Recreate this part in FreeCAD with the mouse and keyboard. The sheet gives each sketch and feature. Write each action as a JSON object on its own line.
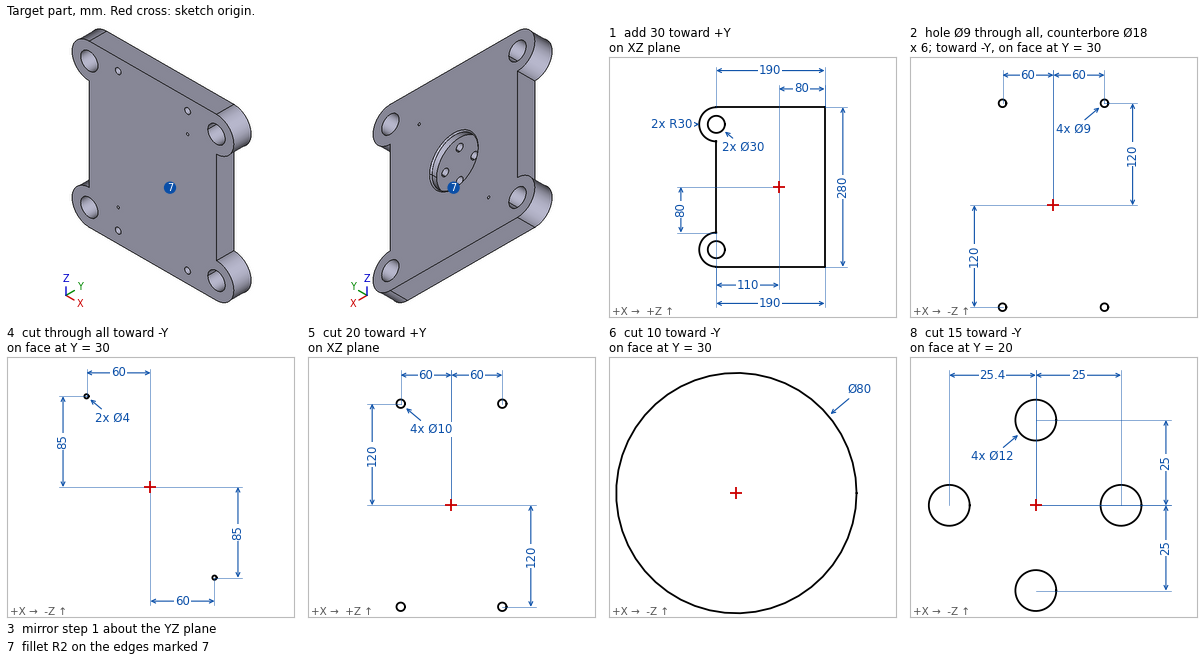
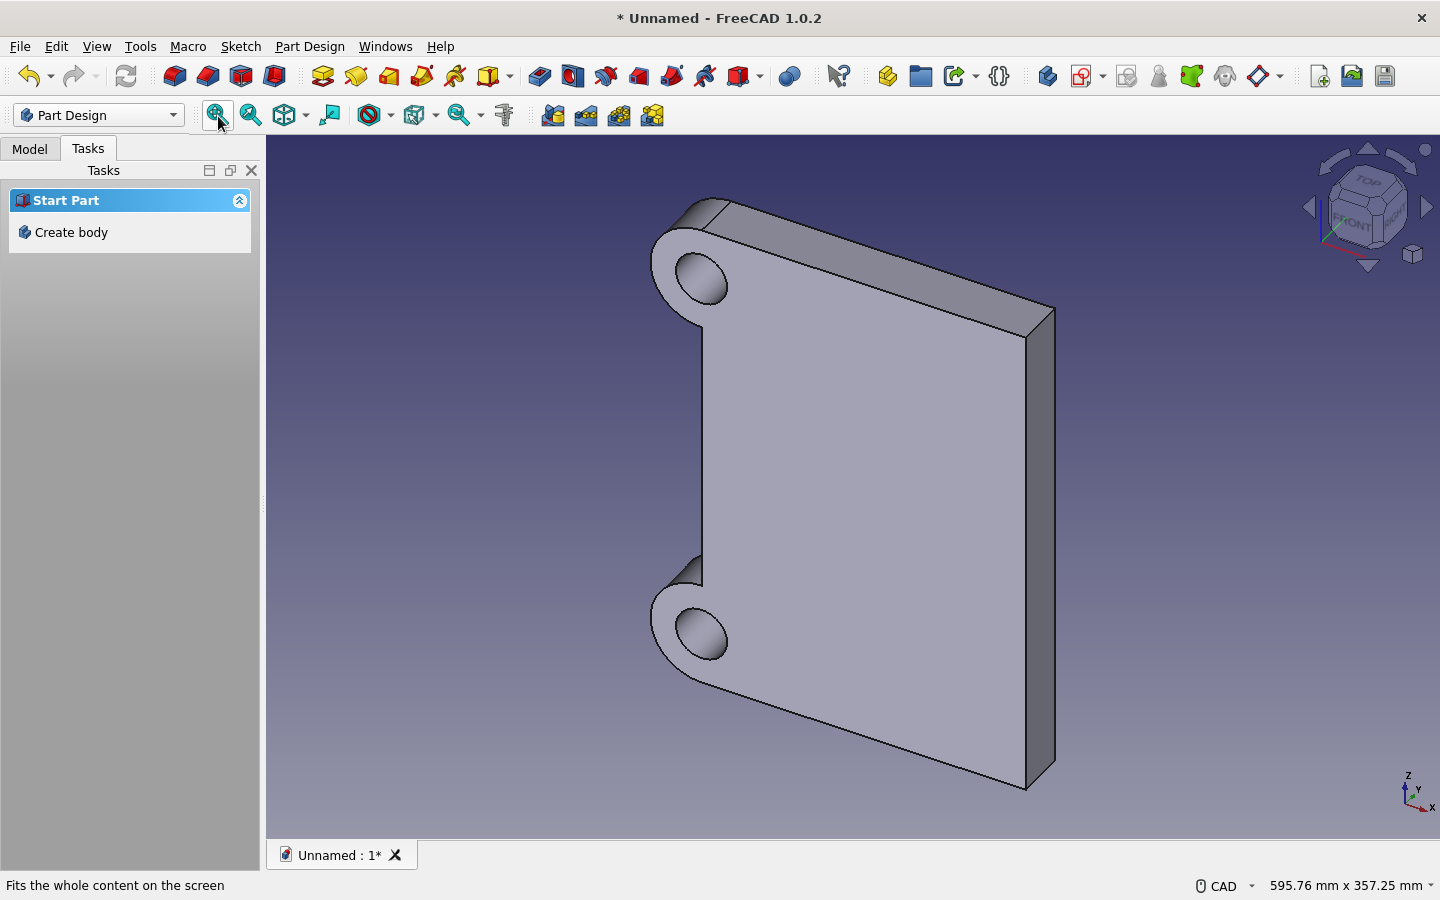
{"action": "key", "text": "4"}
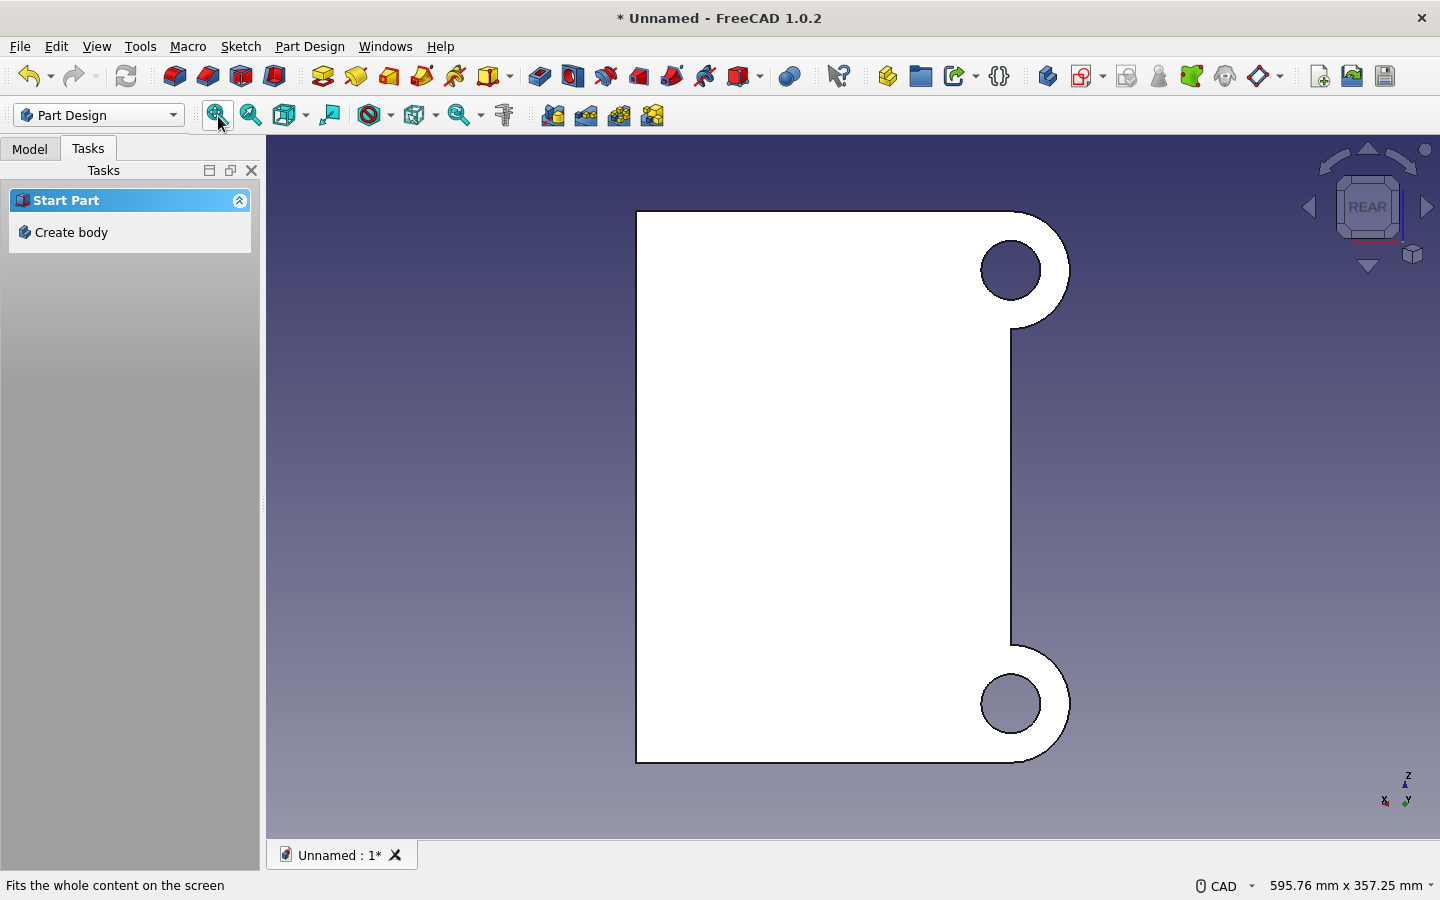
{"action": "left_click", "coordinate": [853, 407]}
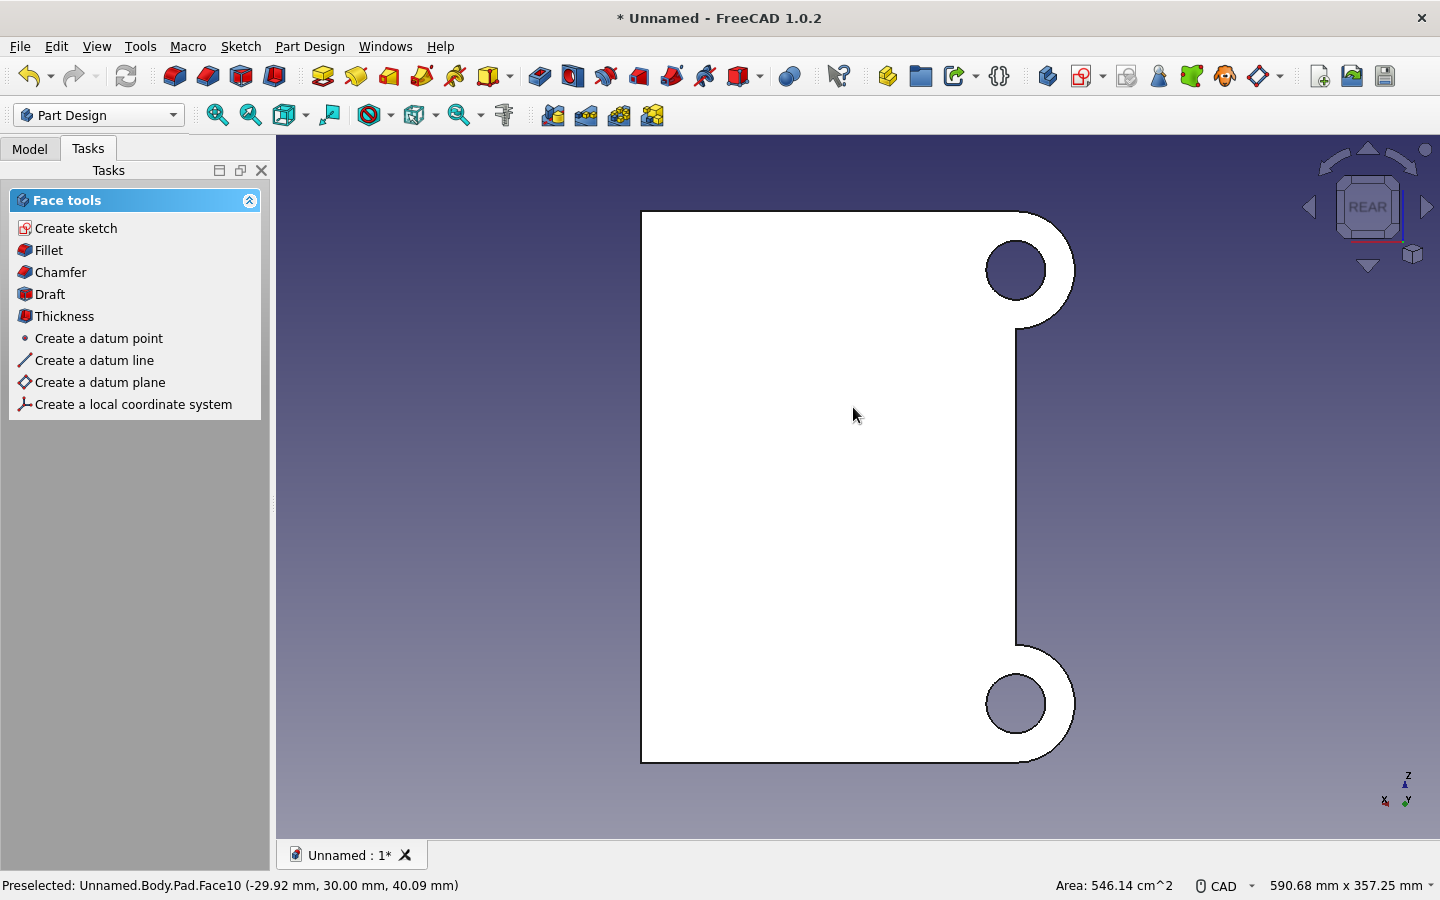
{"action": "left_click", "coordinate": [1080, 76]}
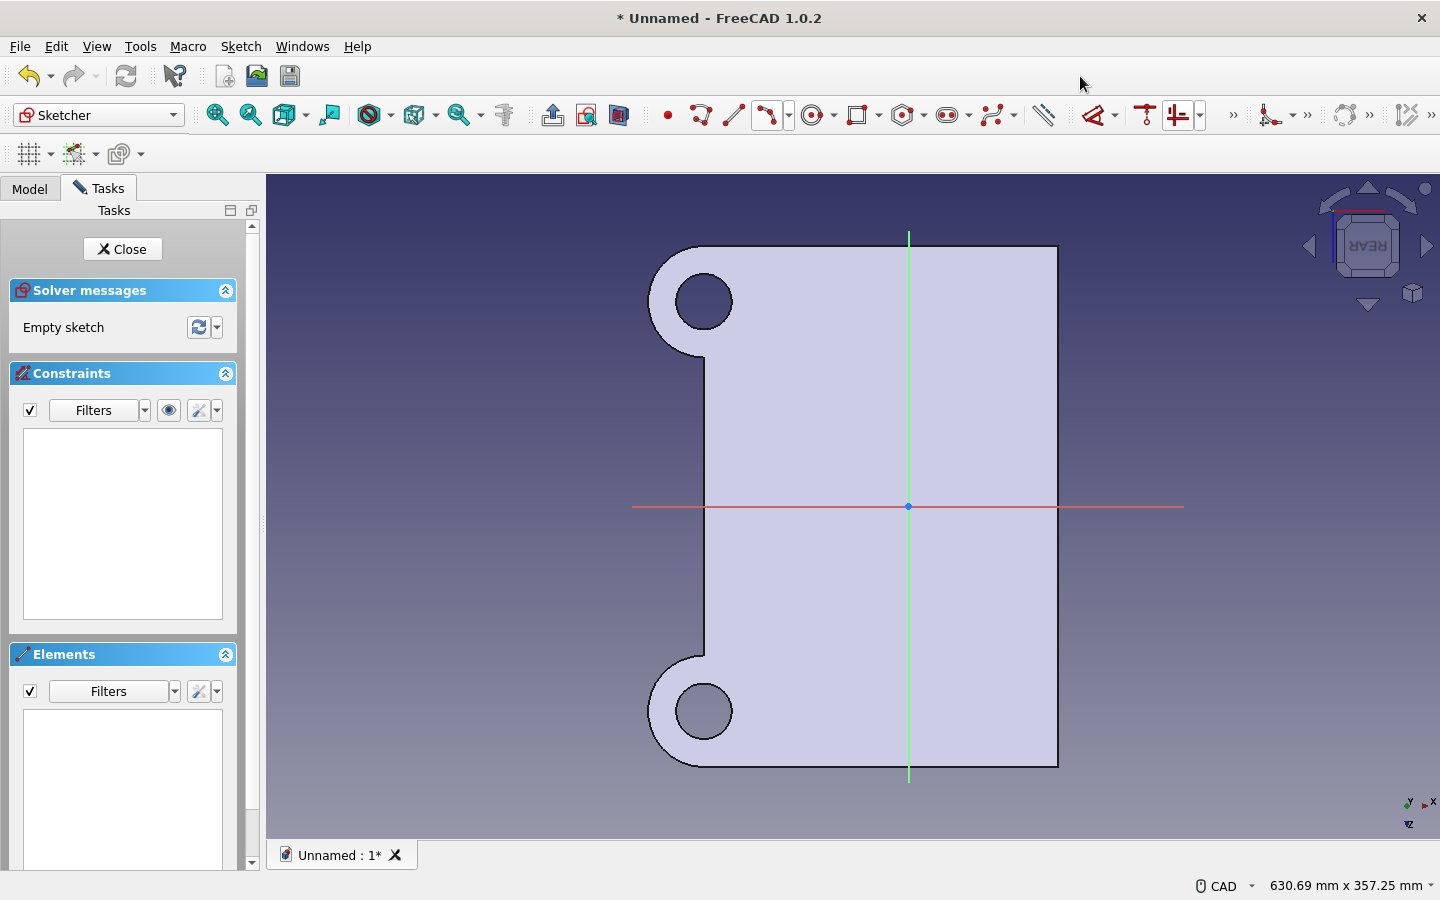
{"action": "left_click", "coordinate": [812, 116]}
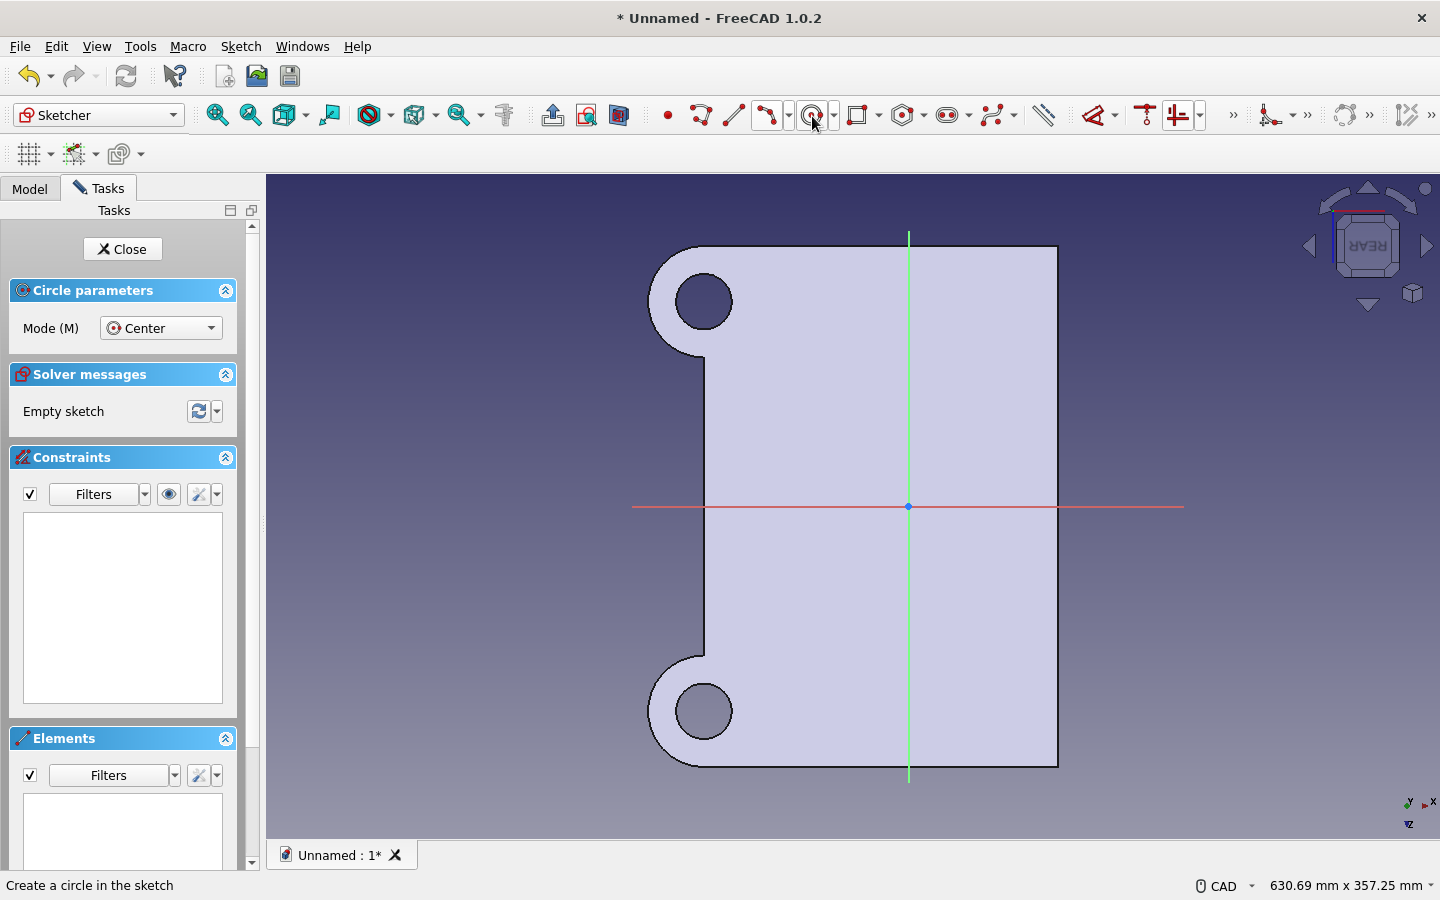
{"action": "scroll", "coordinate": [1020, 283], "scroll_direction": "up", "scroll_amount": 5}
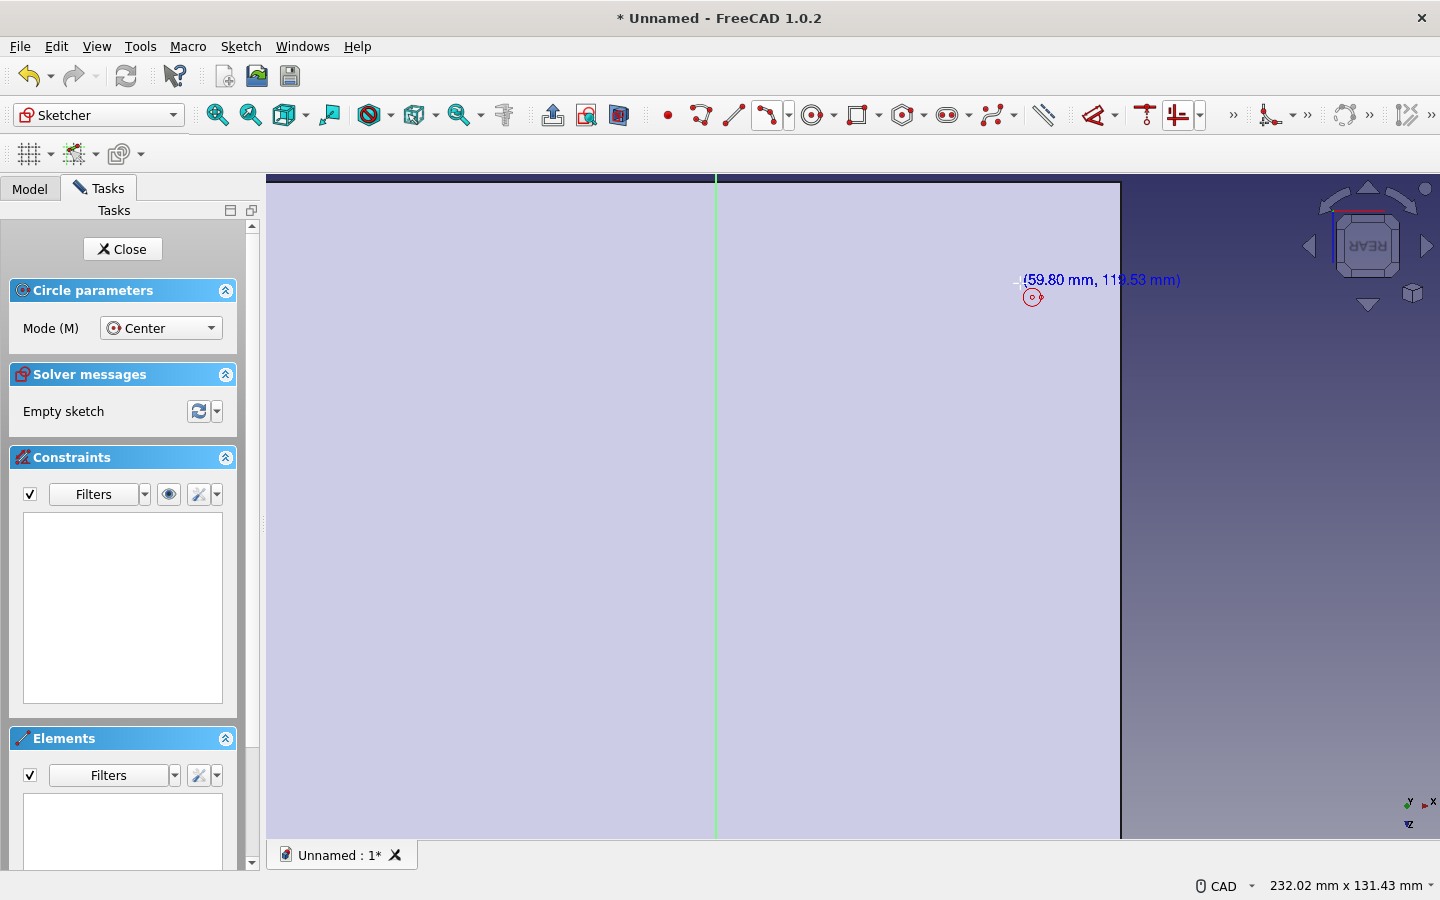
{"action": "left_click", "coordinate": [1020, 283]}
{"action": "mouse_move", "coordinate": [1036, 267]}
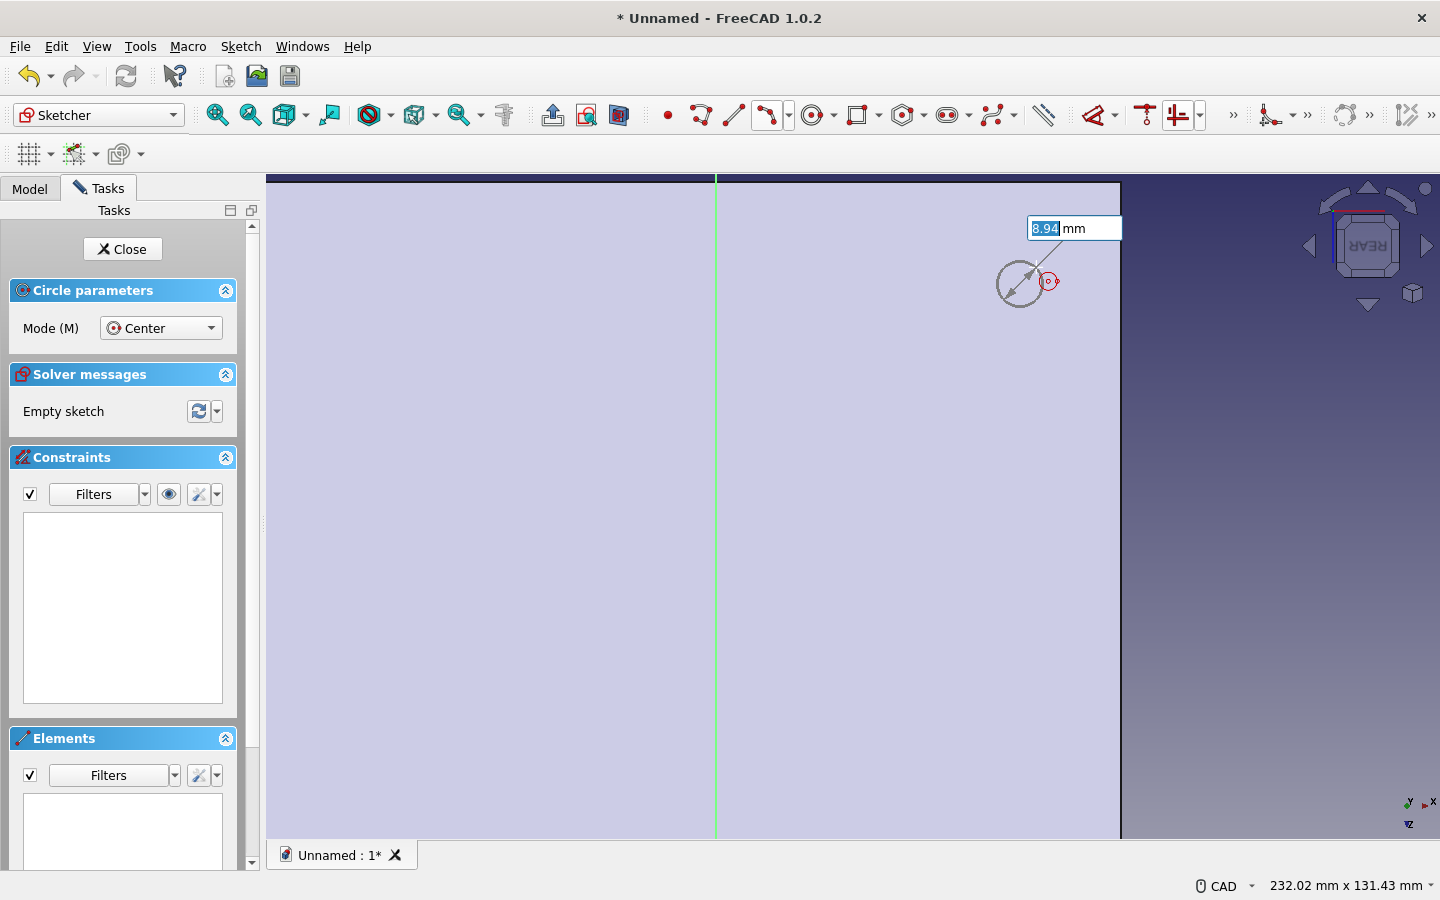
{"action": "type", "text": "9"}
{"action": "key", "text": "Return"}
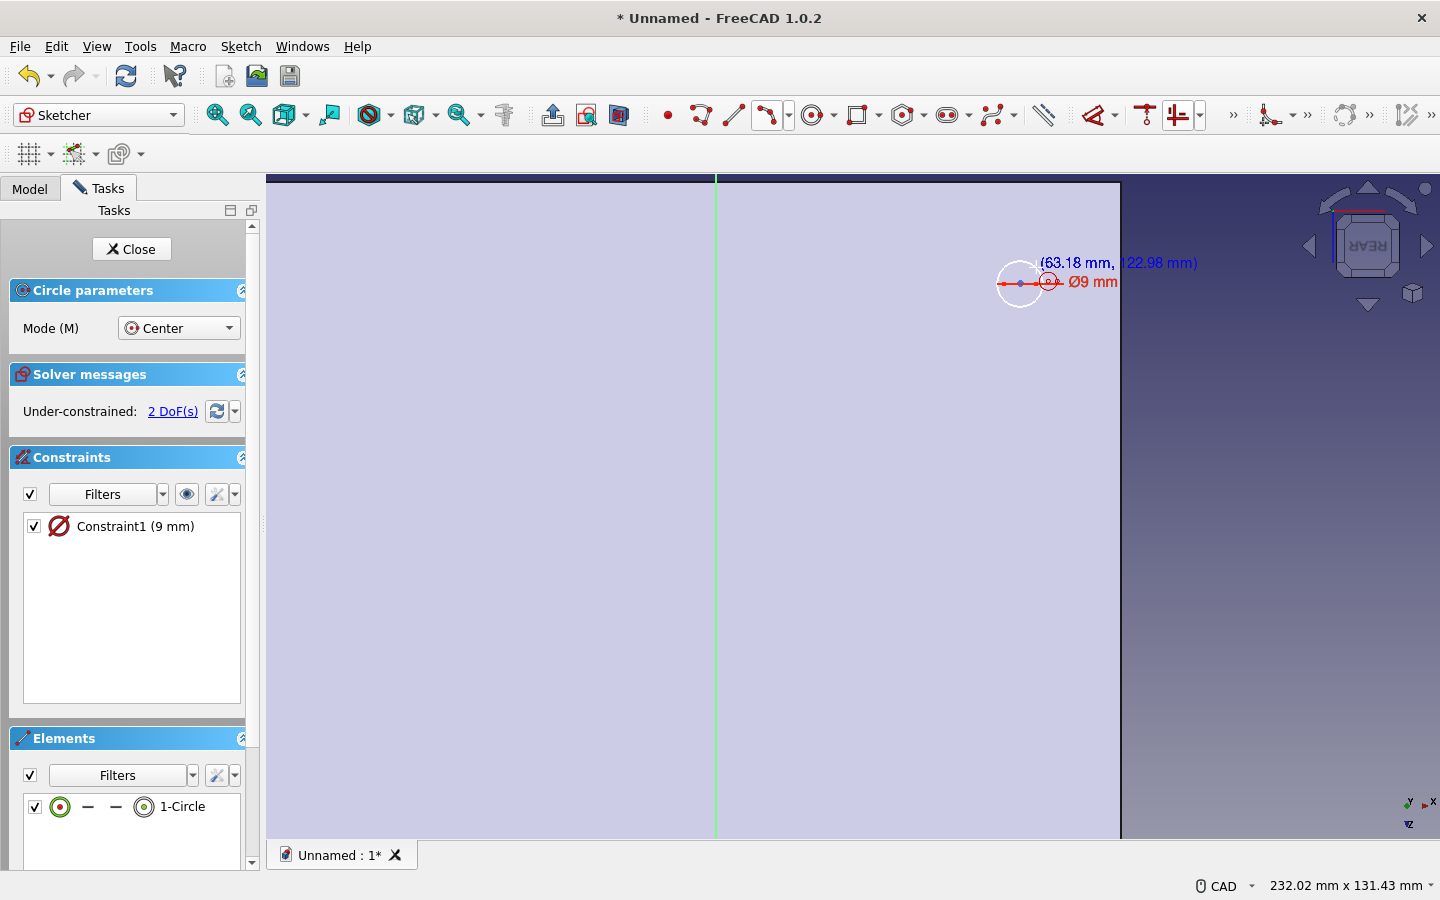
{"action": "left_click", "coordinate": [413, 283]}
{"action": "mouse_move", "coordinate": [429, 267]}